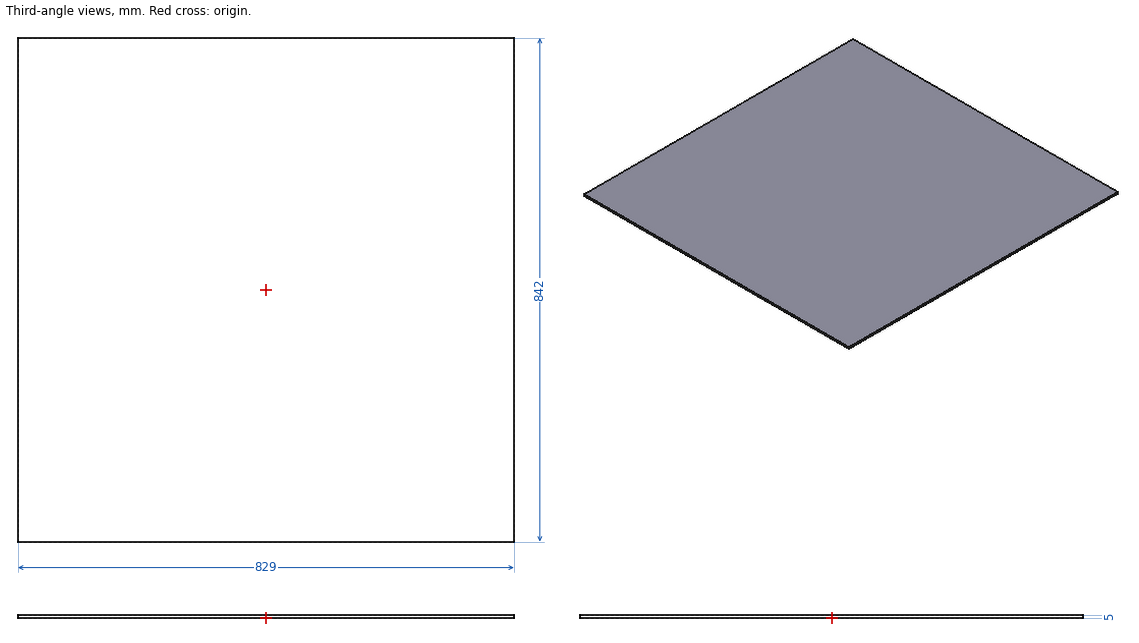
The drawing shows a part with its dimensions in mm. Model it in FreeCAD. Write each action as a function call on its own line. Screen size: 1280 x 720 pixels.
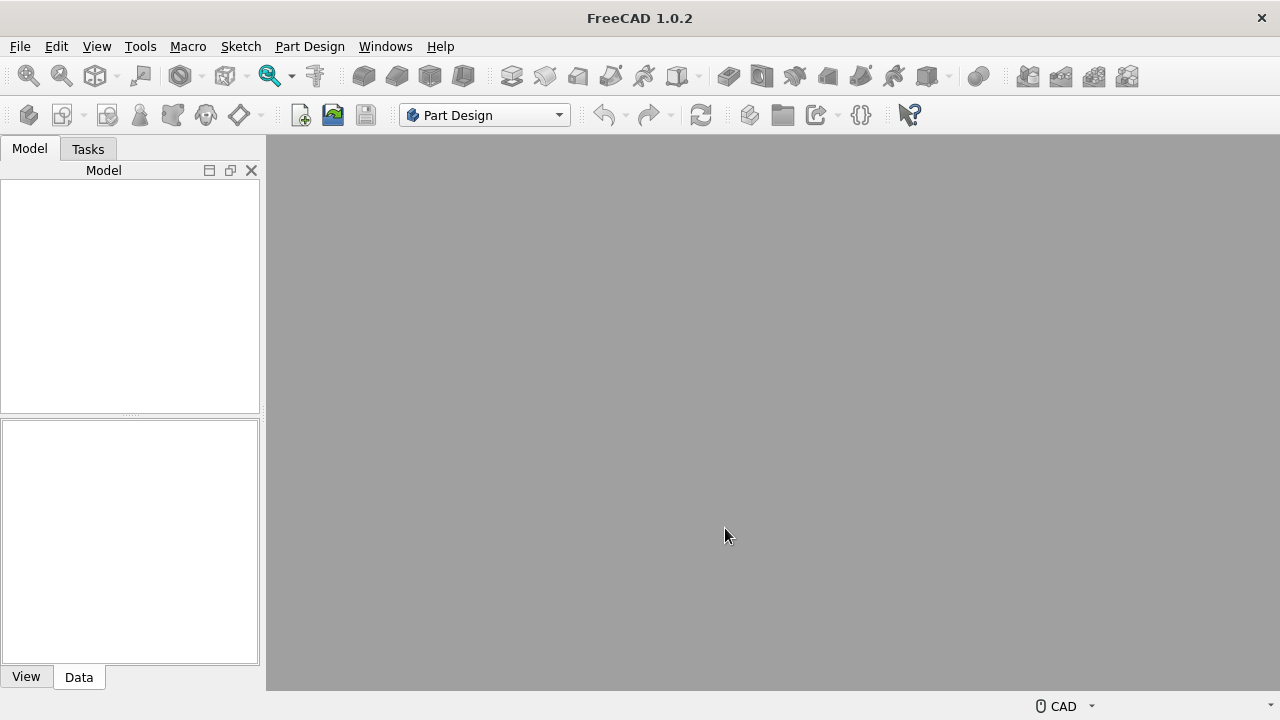
key(ctrl+n)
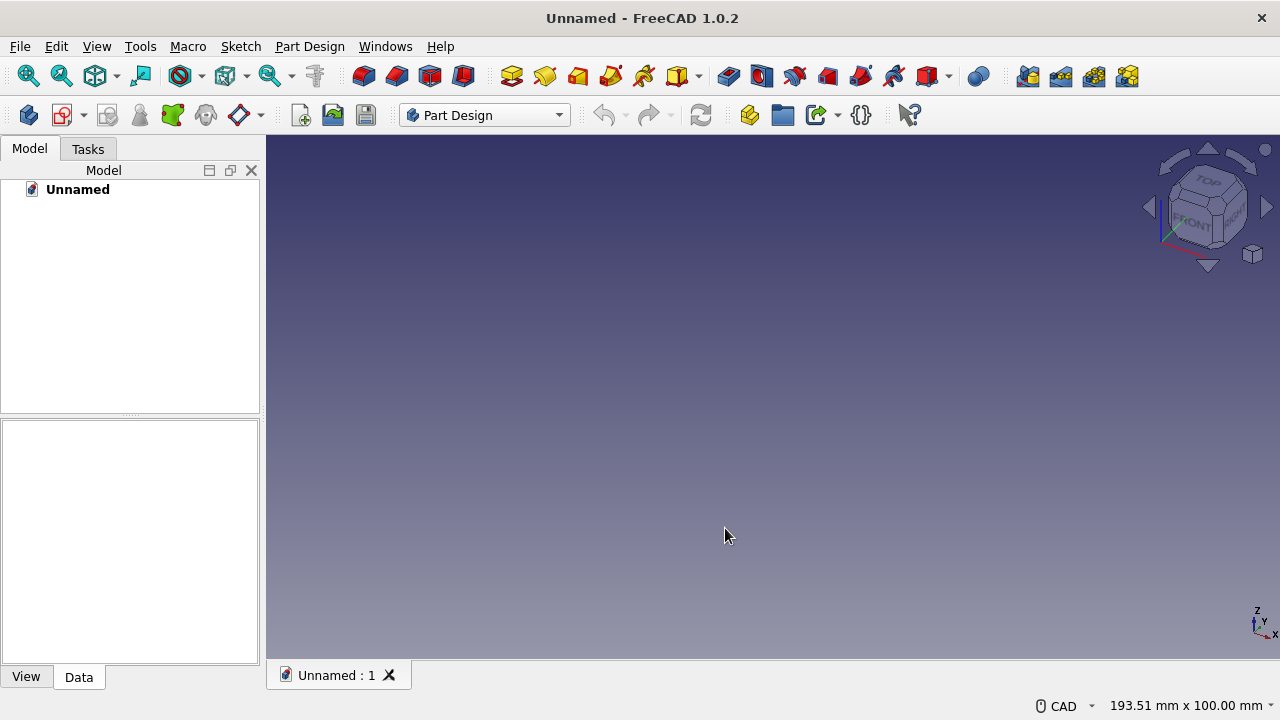
click(62, 116)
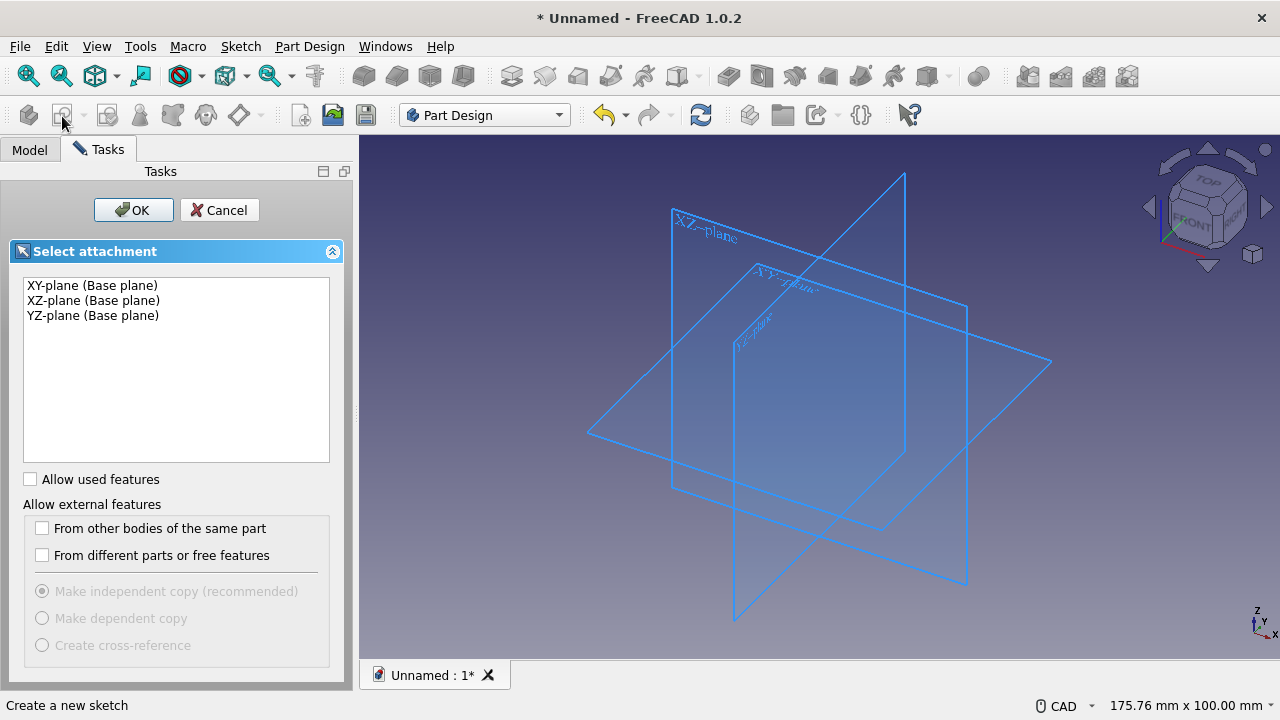
click(84, 286)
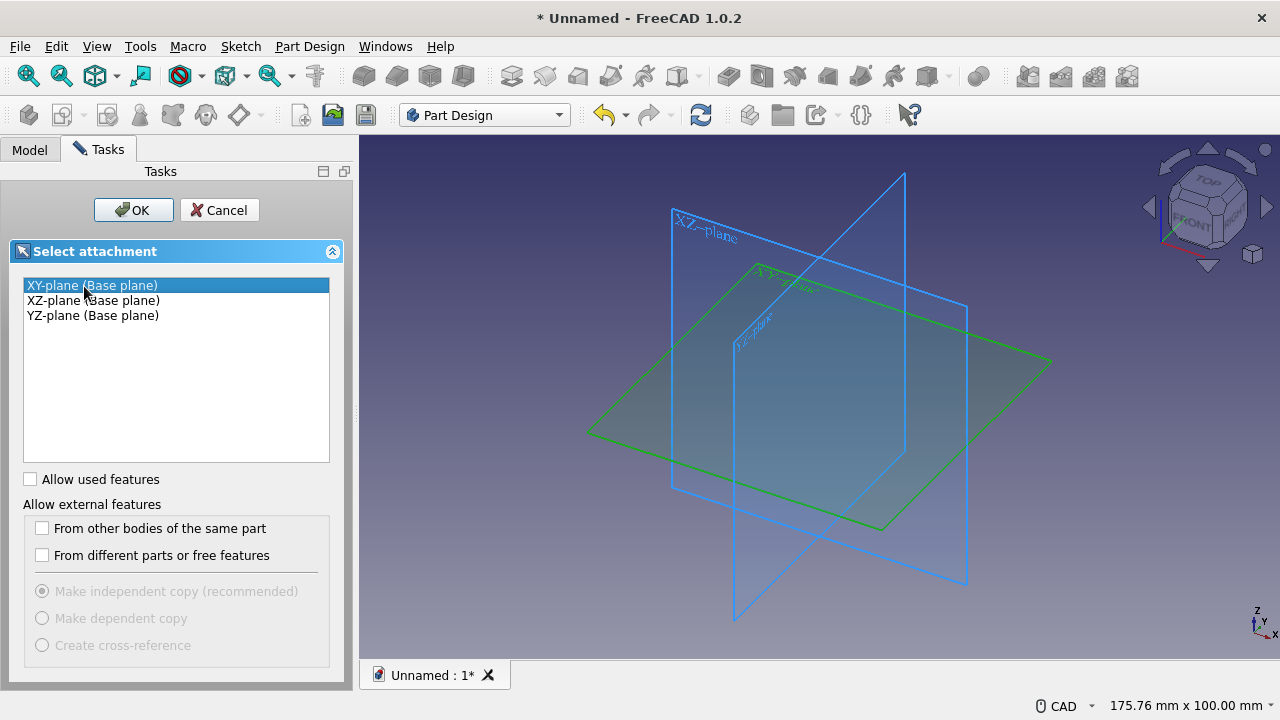
click(134, 210)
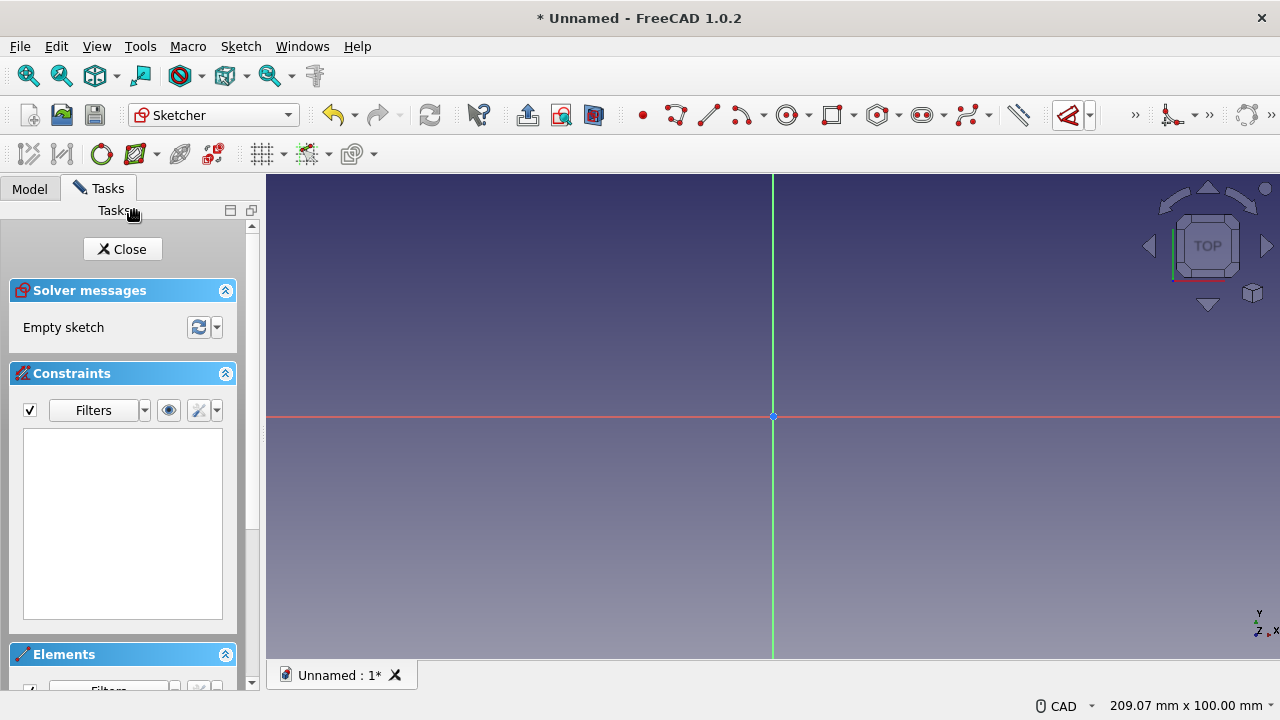
scroll(699, 416, down, 13)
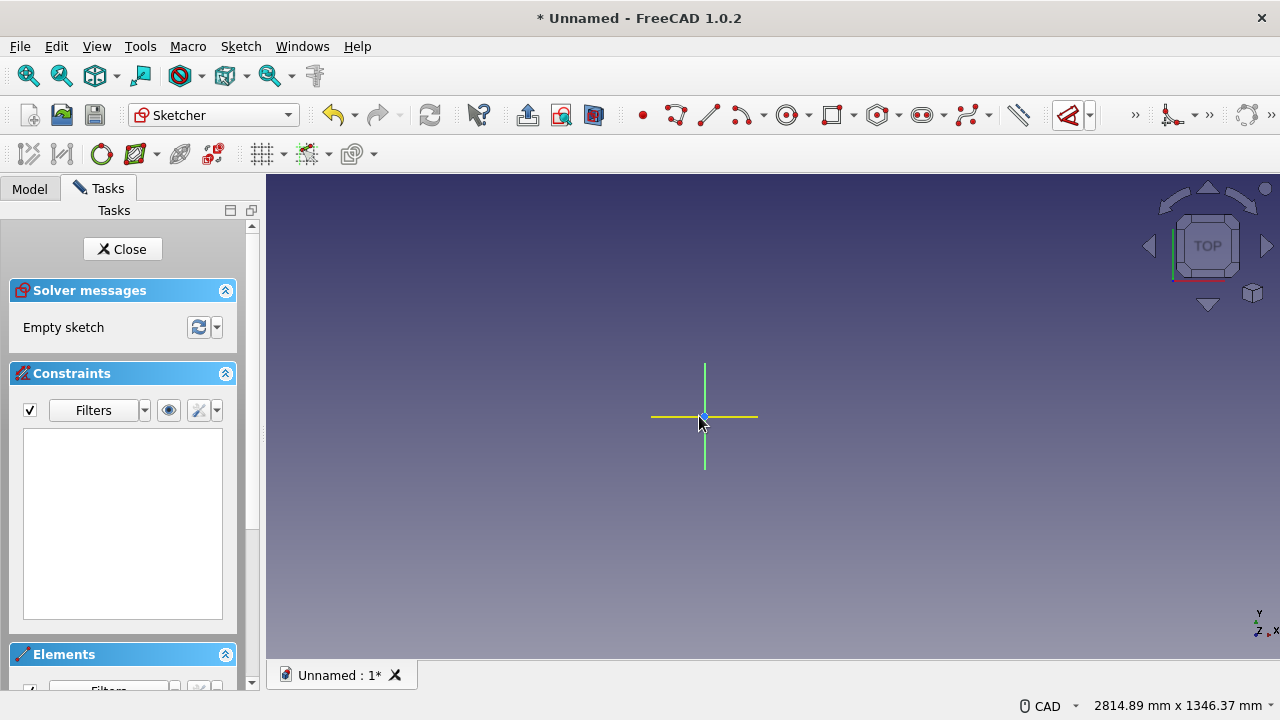
key(g)
key(v)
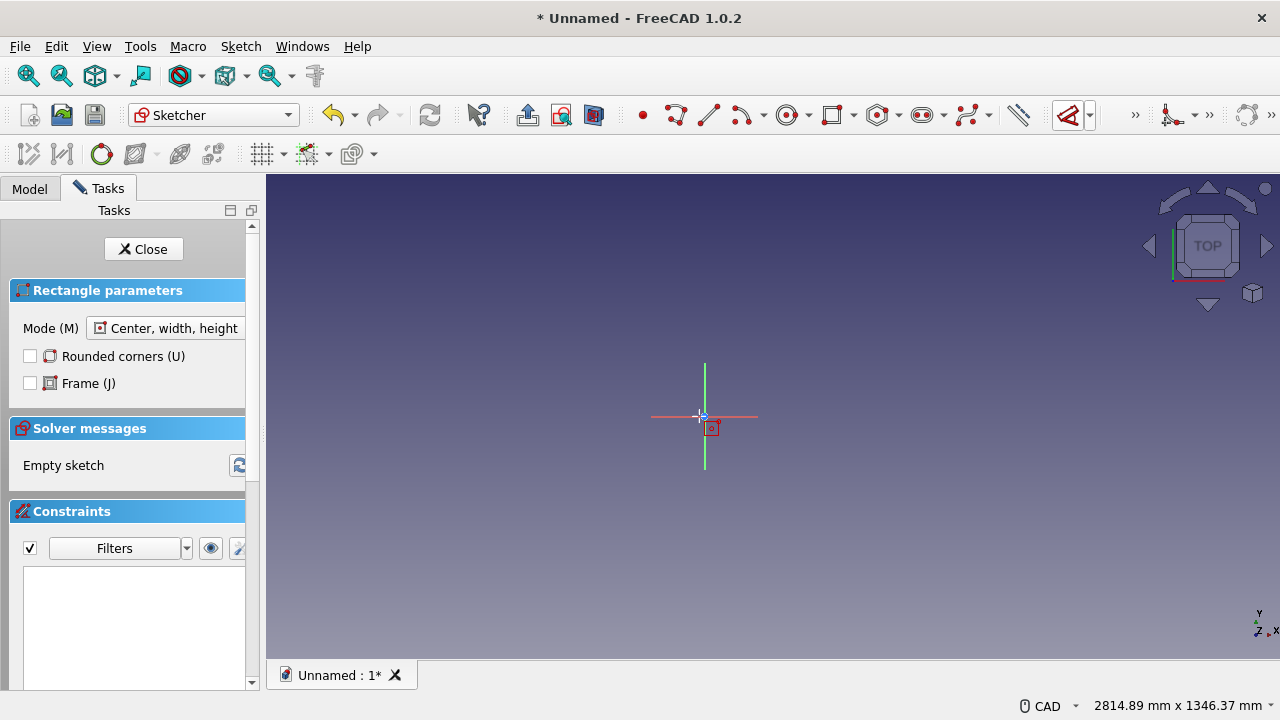
click(705, 416)
click(854, 265)
key(Escape)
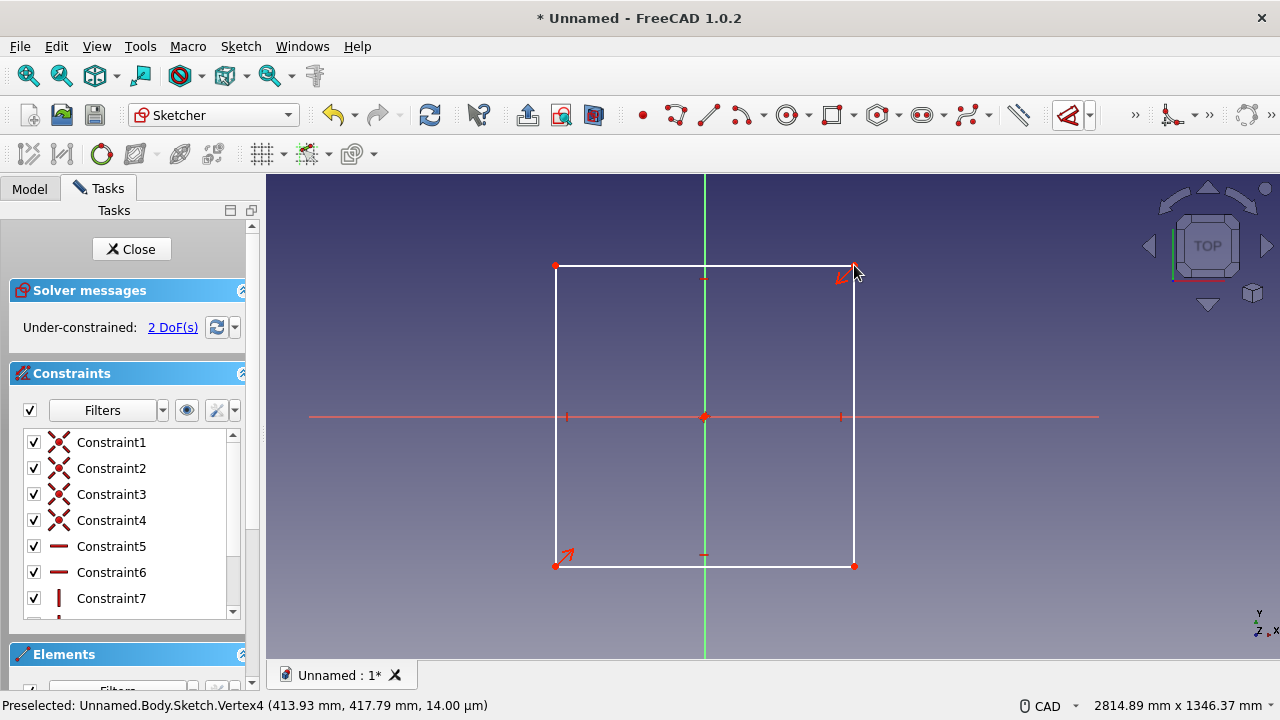
key(d)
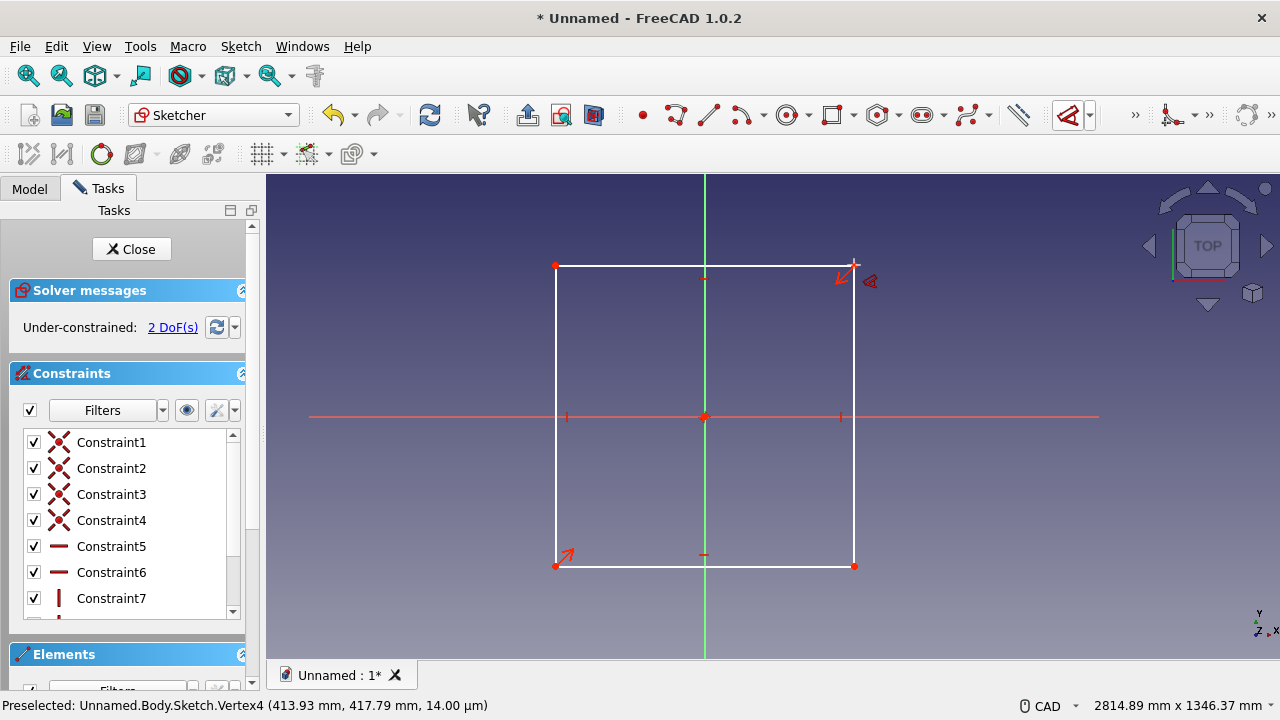
click(645, 567)
click(636, 601)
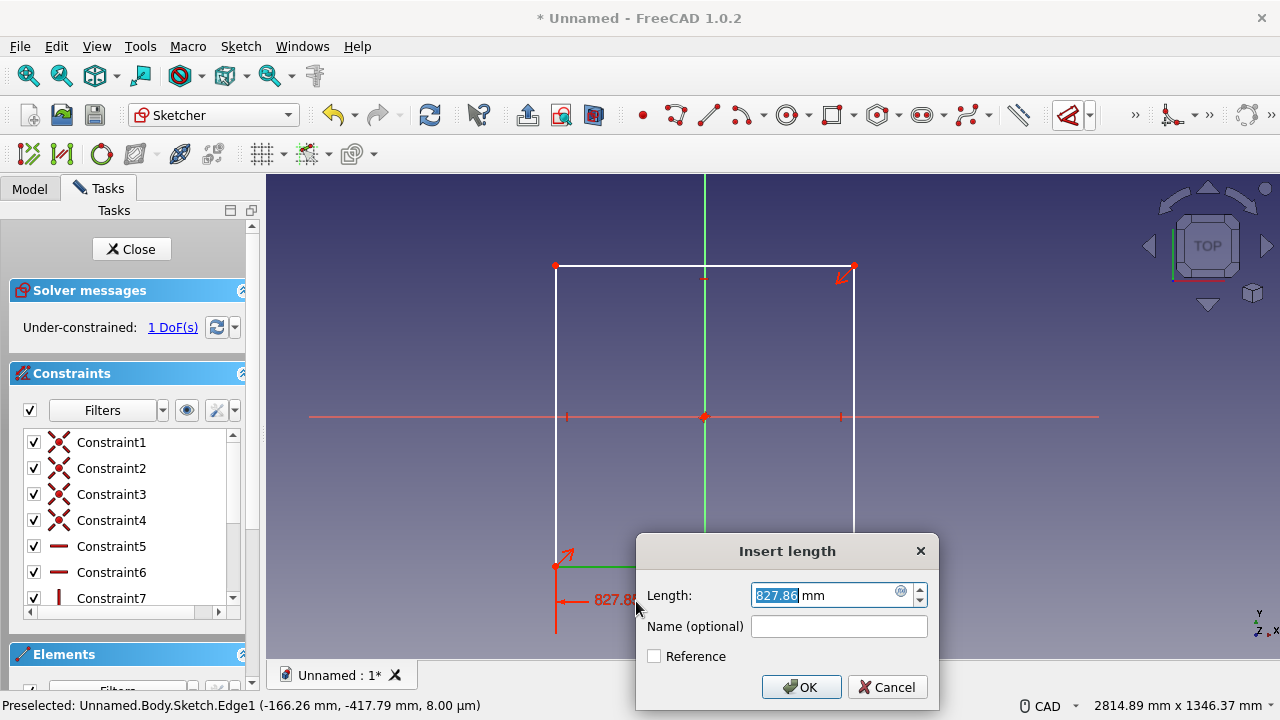
text(829)
key(Return)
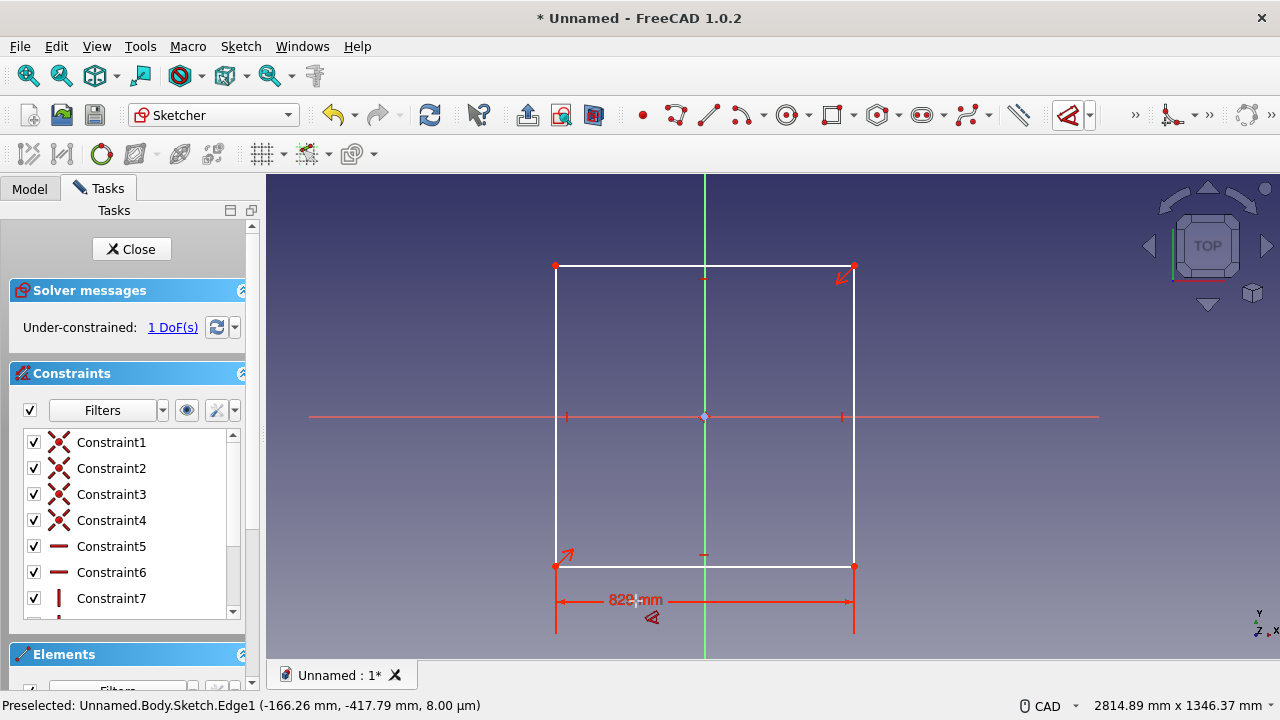
click(854, 477)
click(888, 347)